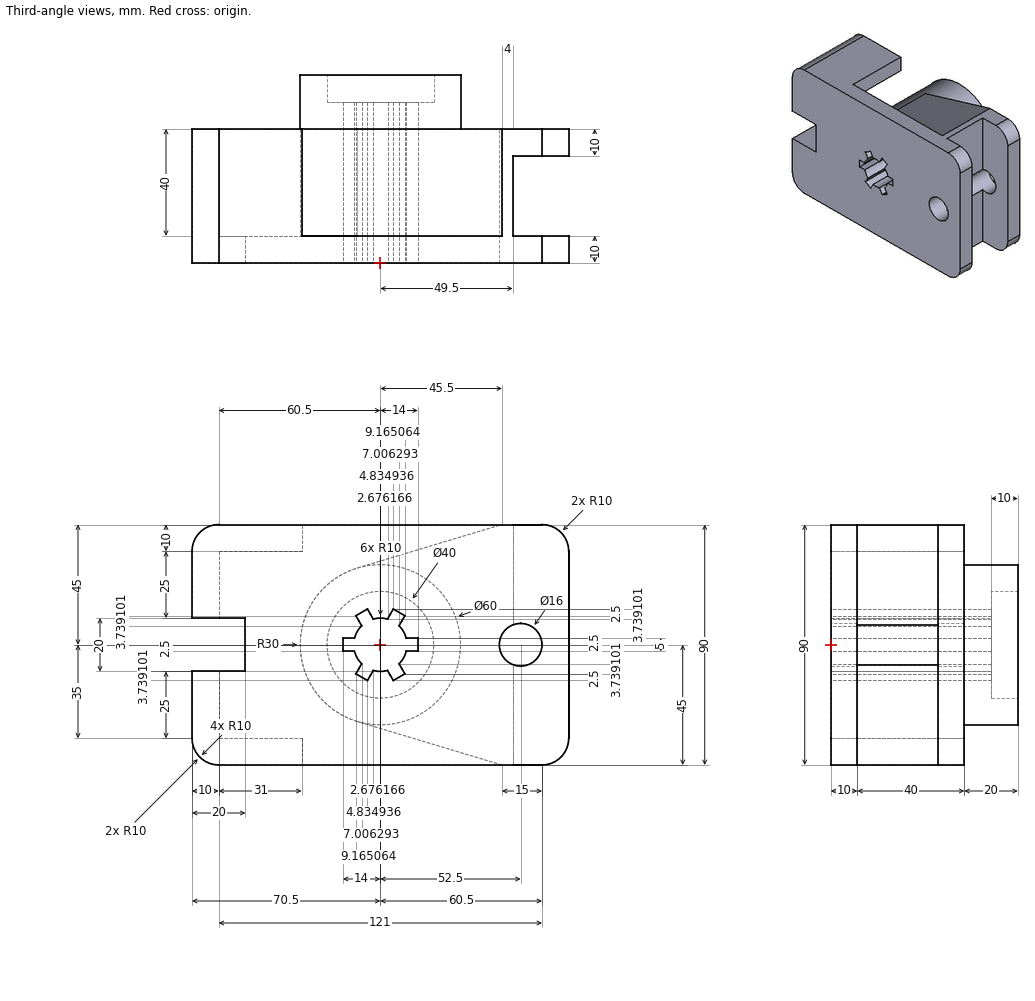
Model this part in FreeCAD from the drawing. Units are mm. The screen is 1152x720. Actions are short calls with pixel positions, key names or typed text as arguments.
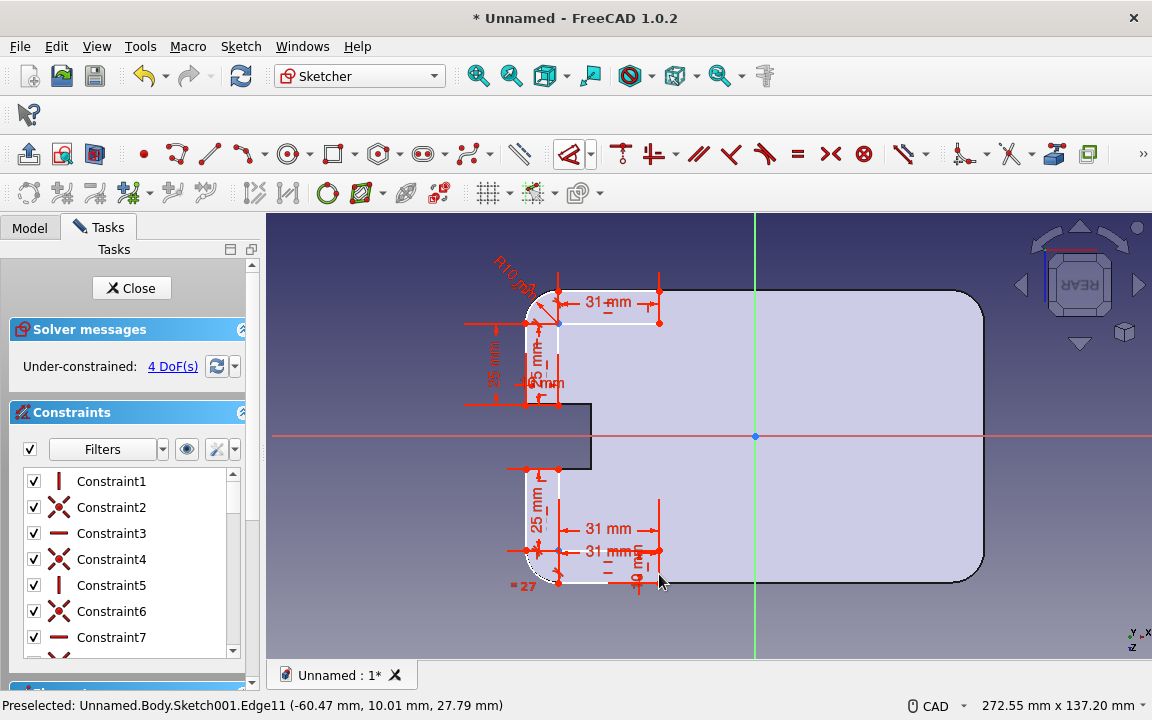
click(526, 324)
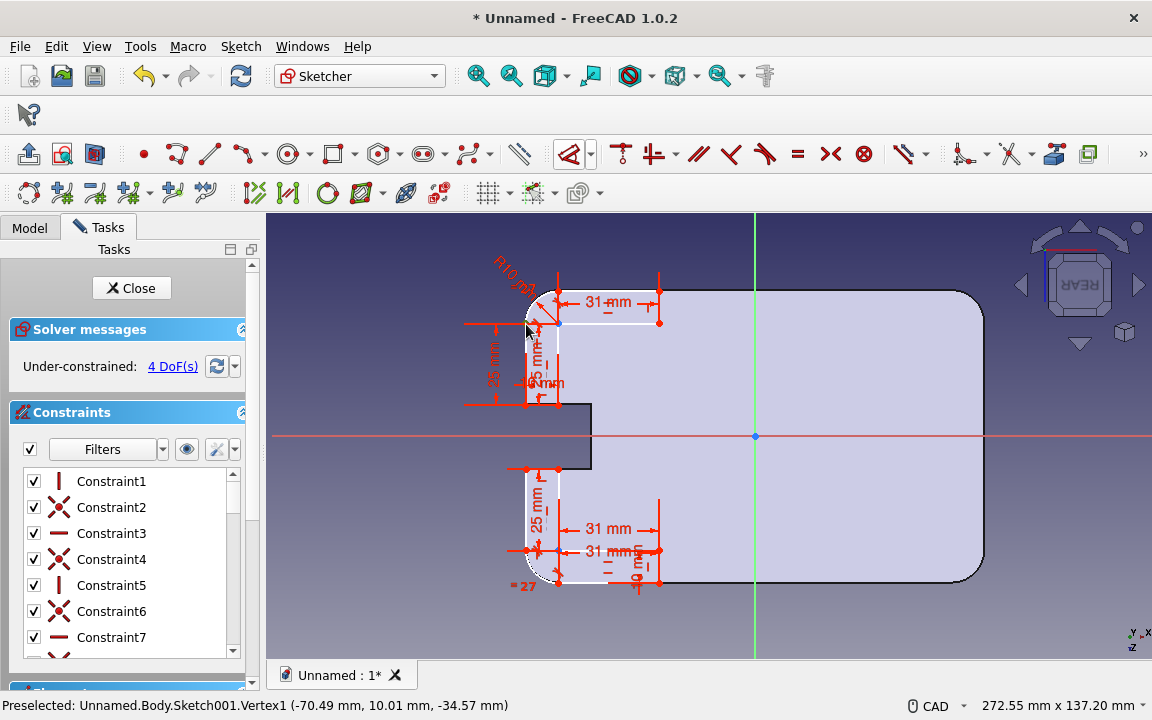
key(i)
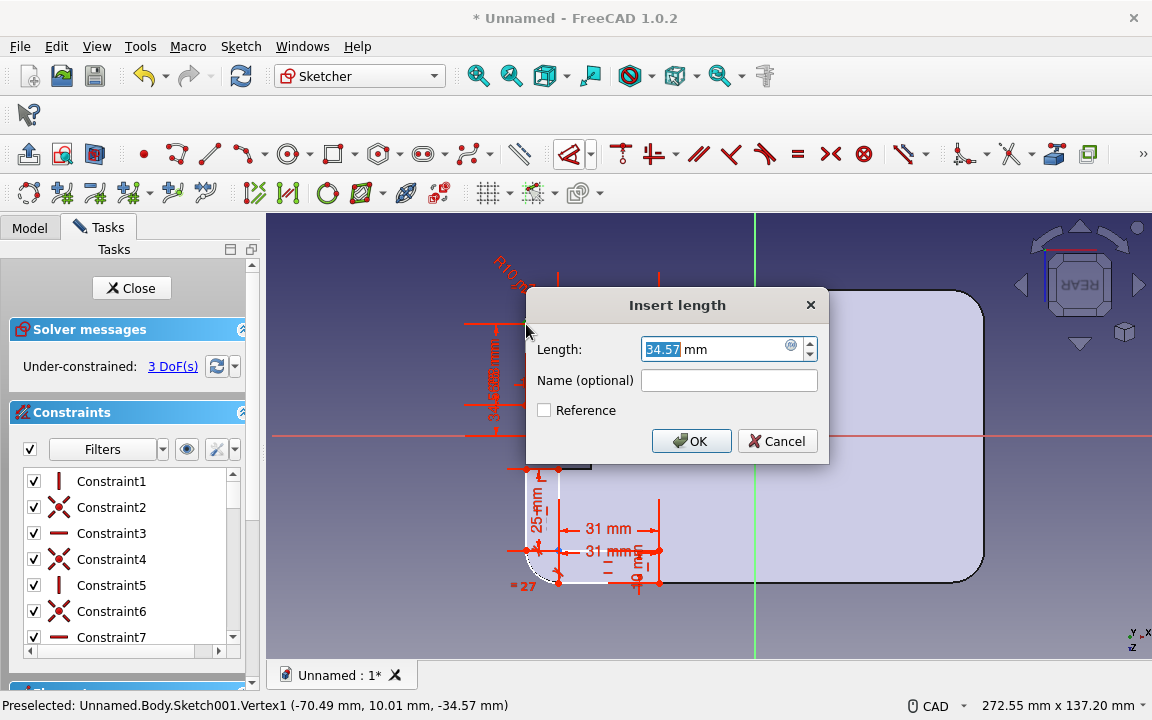
text(35)
key(Return)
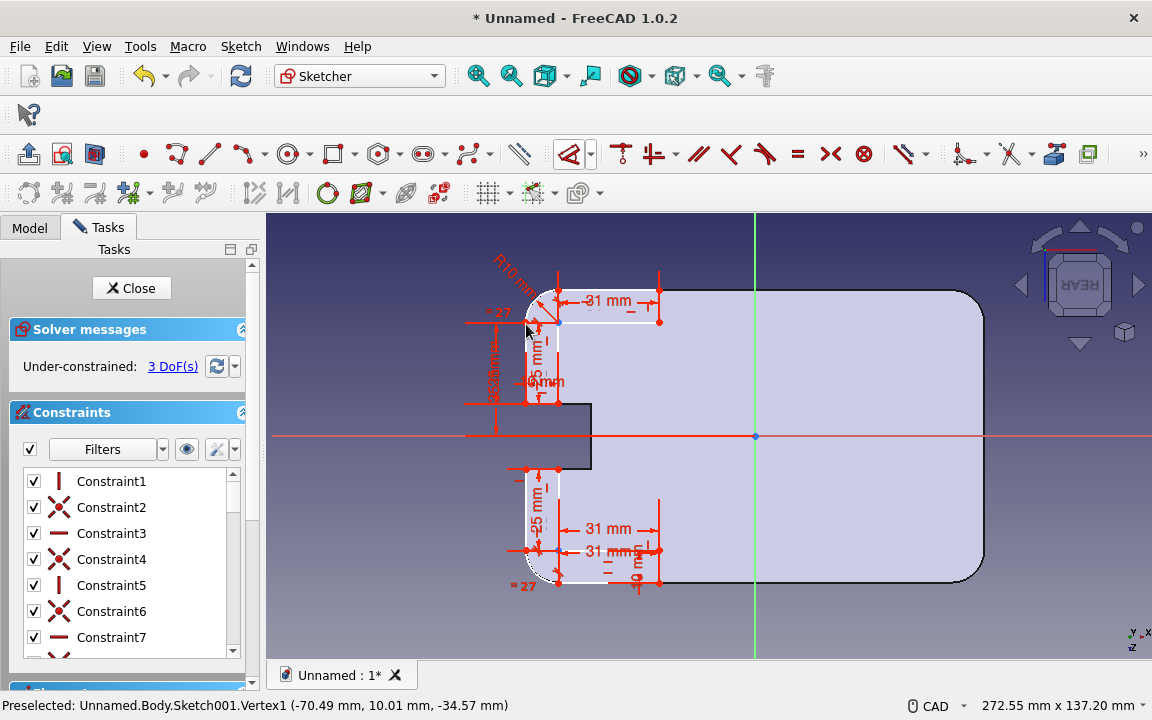
click(559, 583)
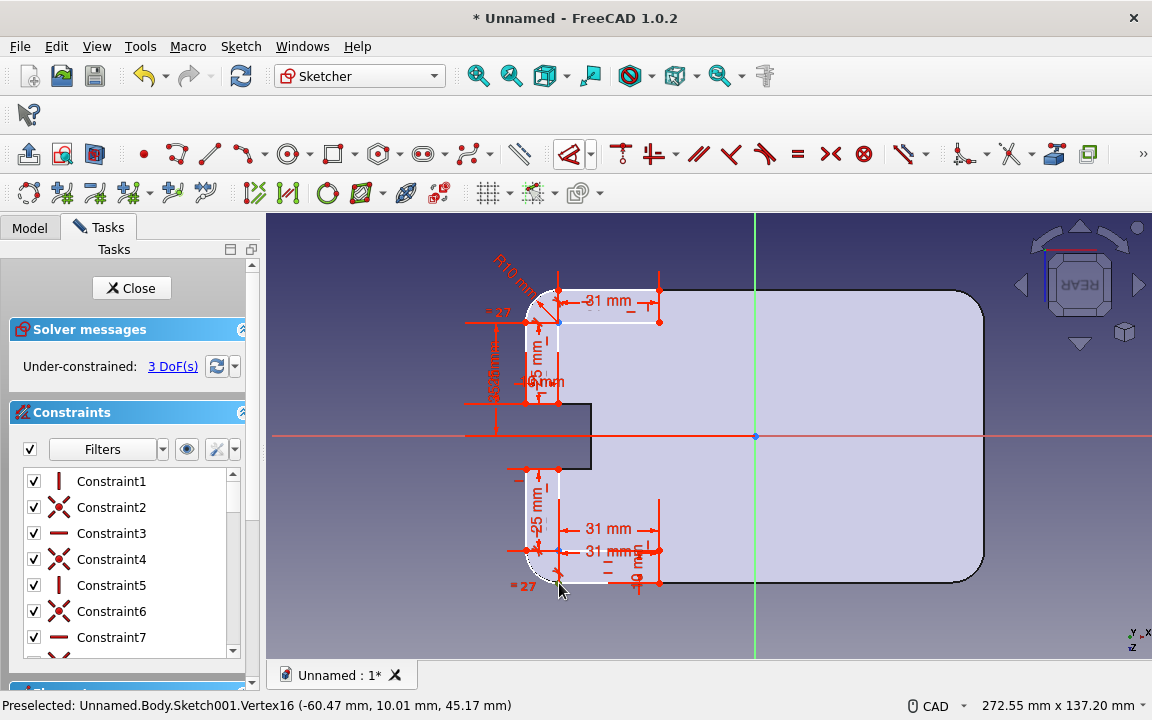
key(i)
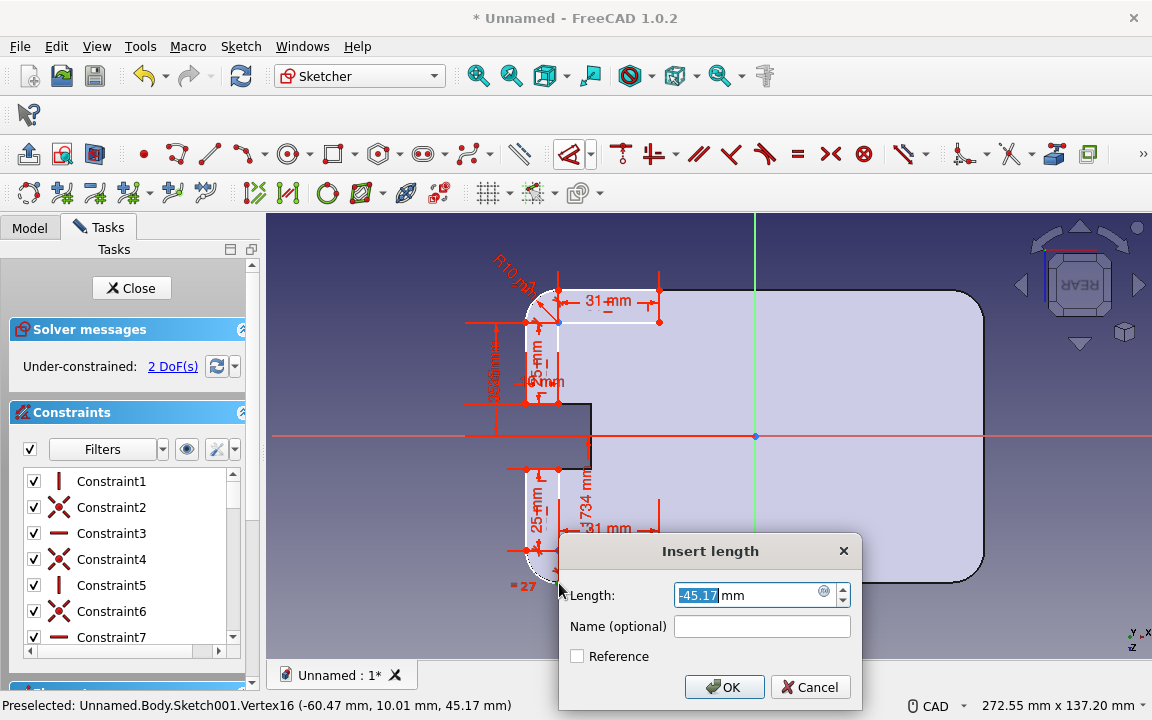
text(-45)
key(Return)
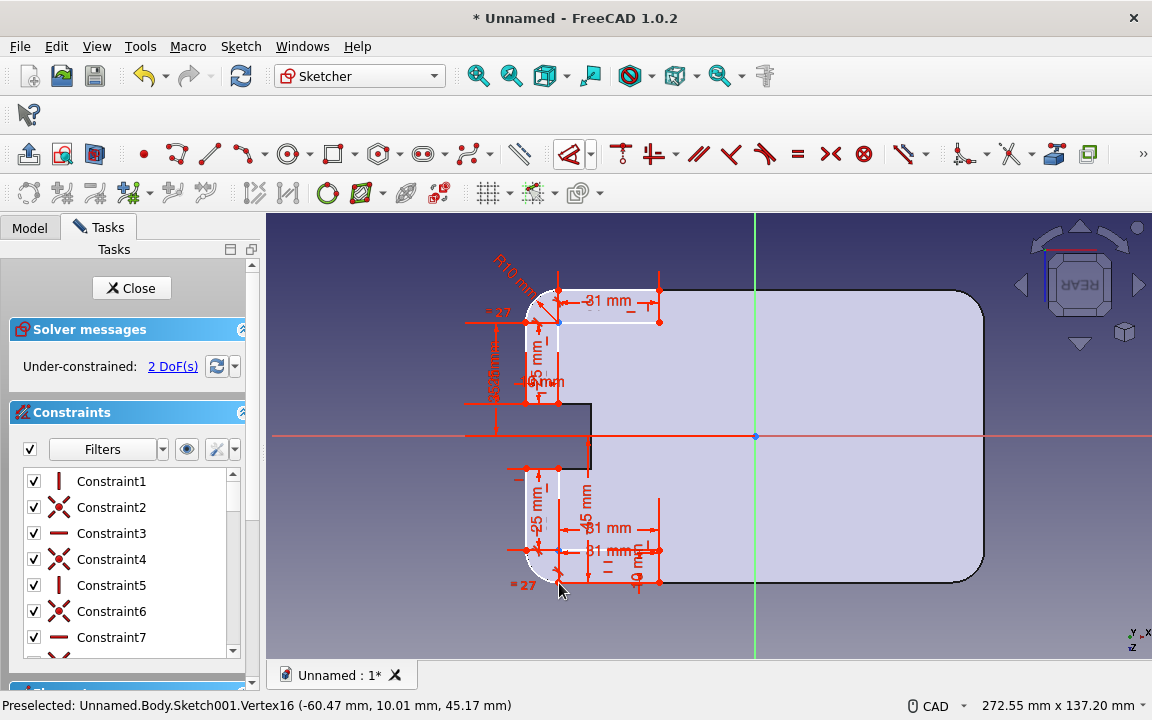
click(526, 323)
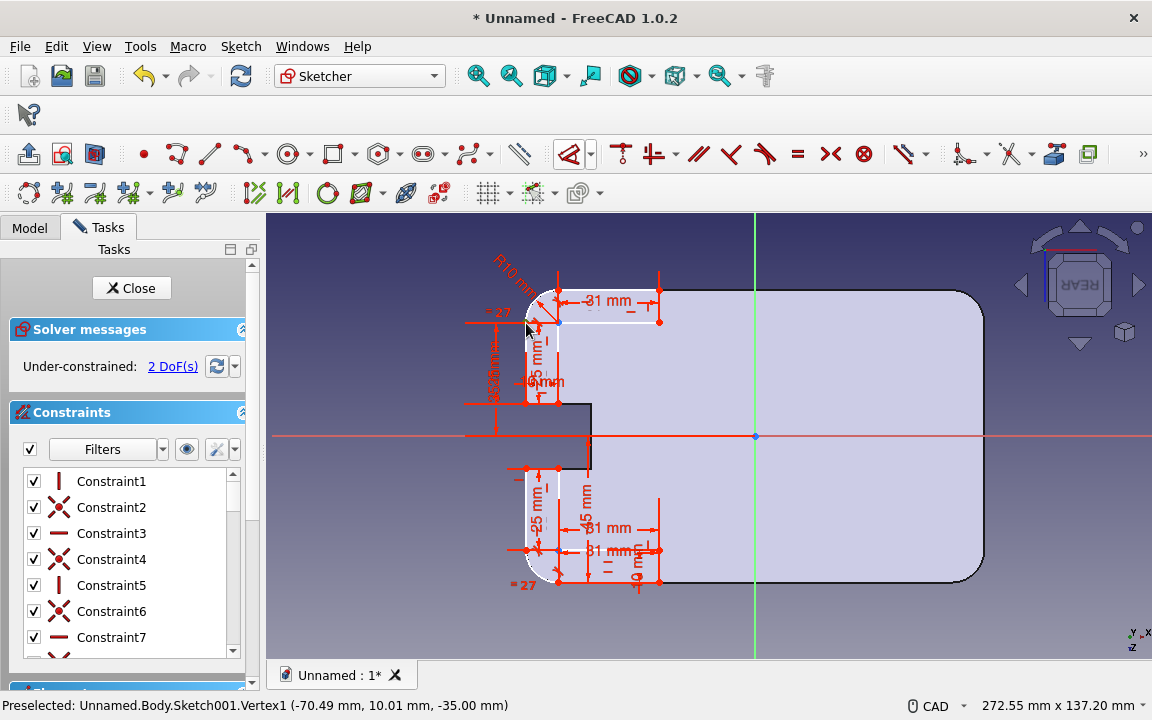
click(590, 154)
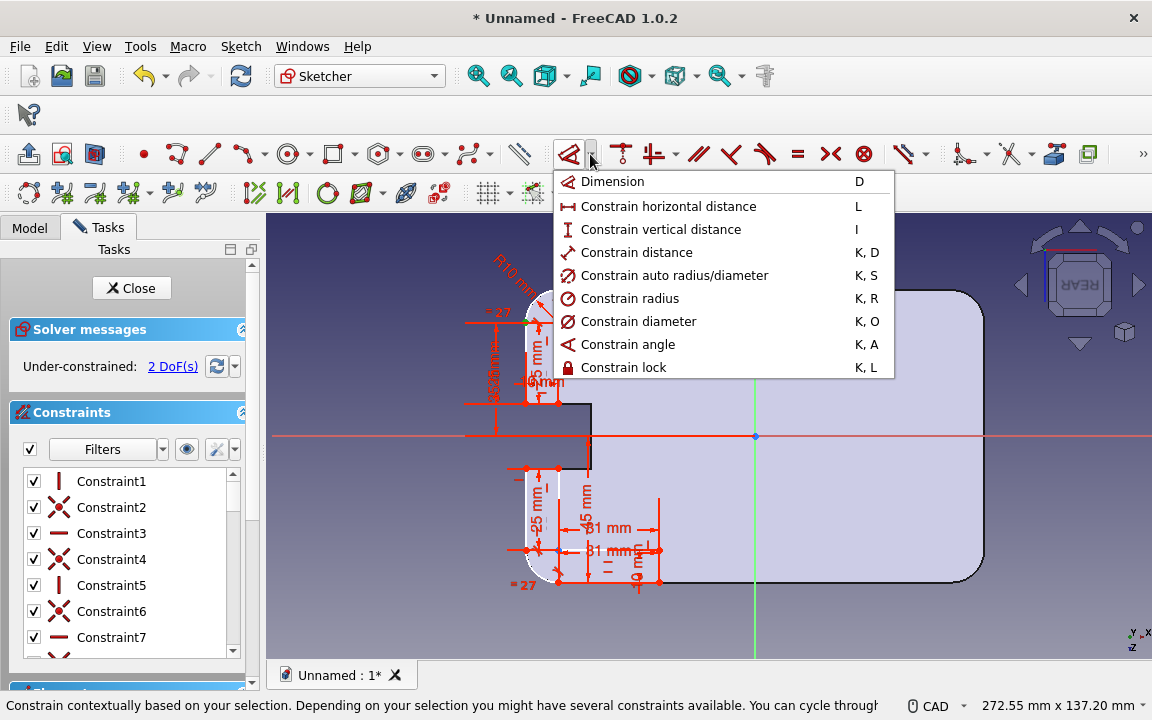
click(724, 206)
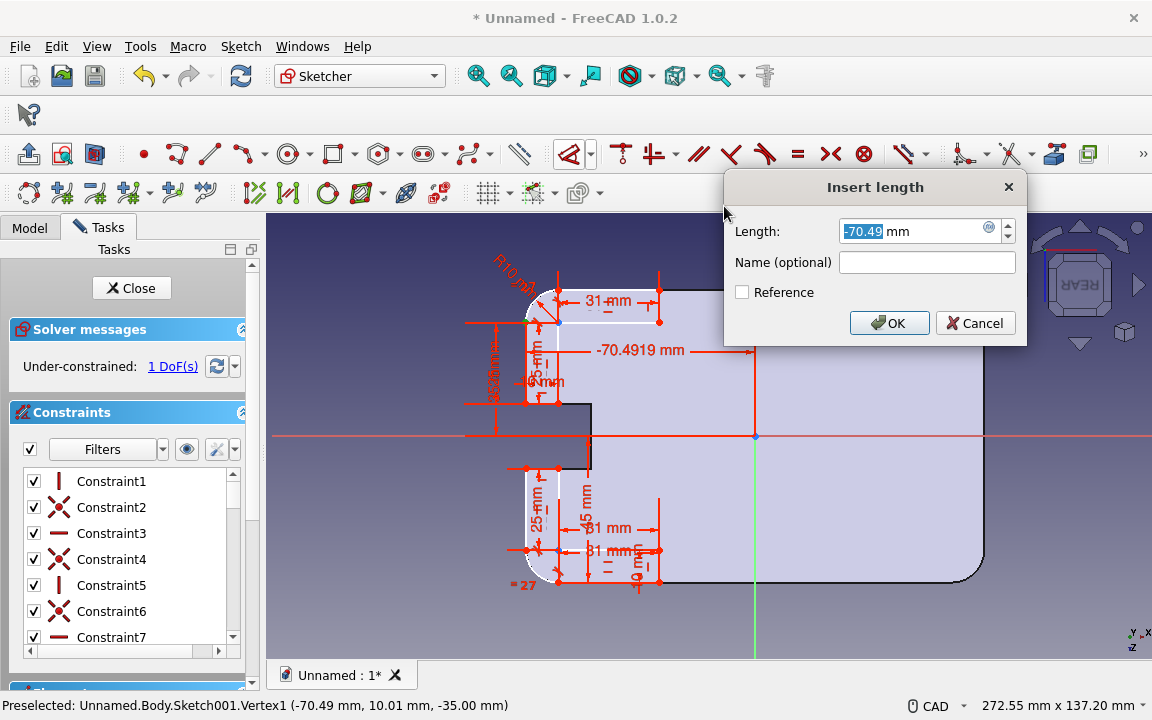
text(-70.5)
key(Return)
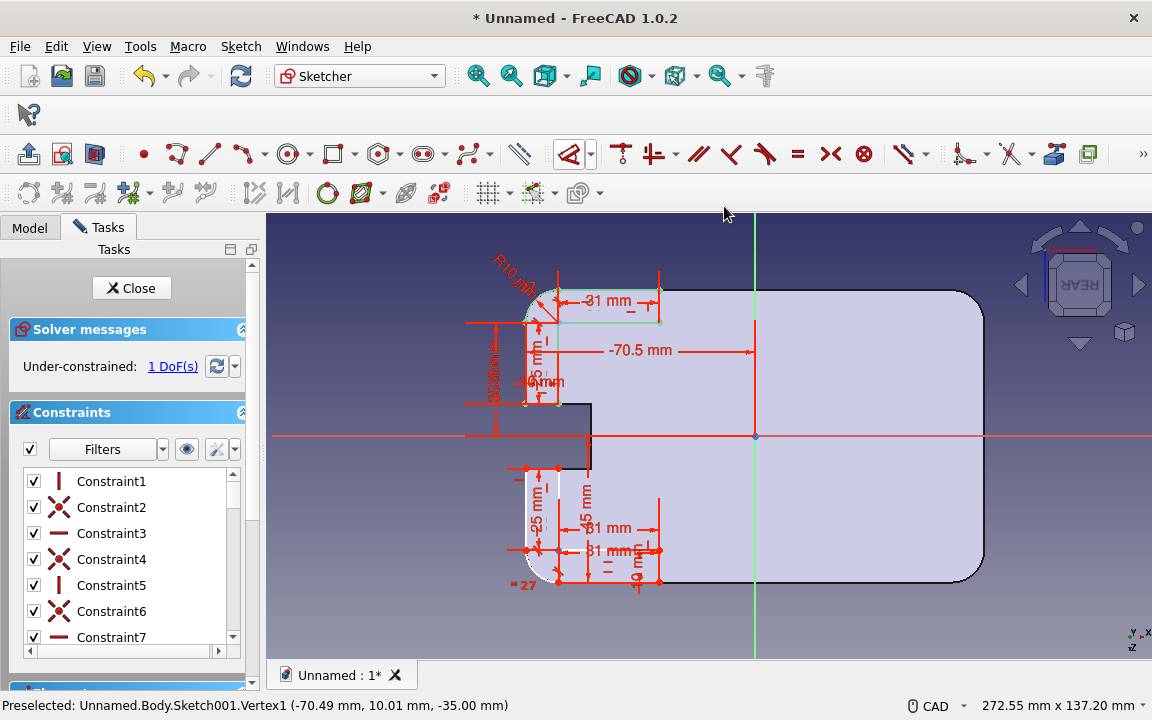
click(559, 583)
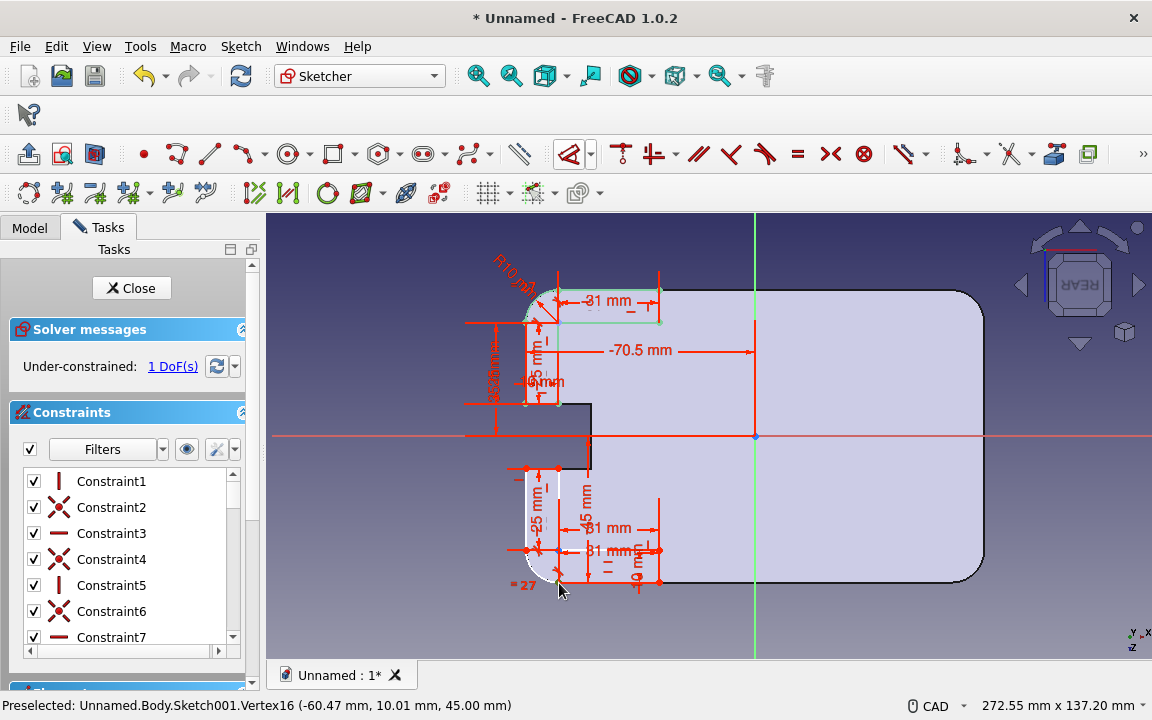
key(l)